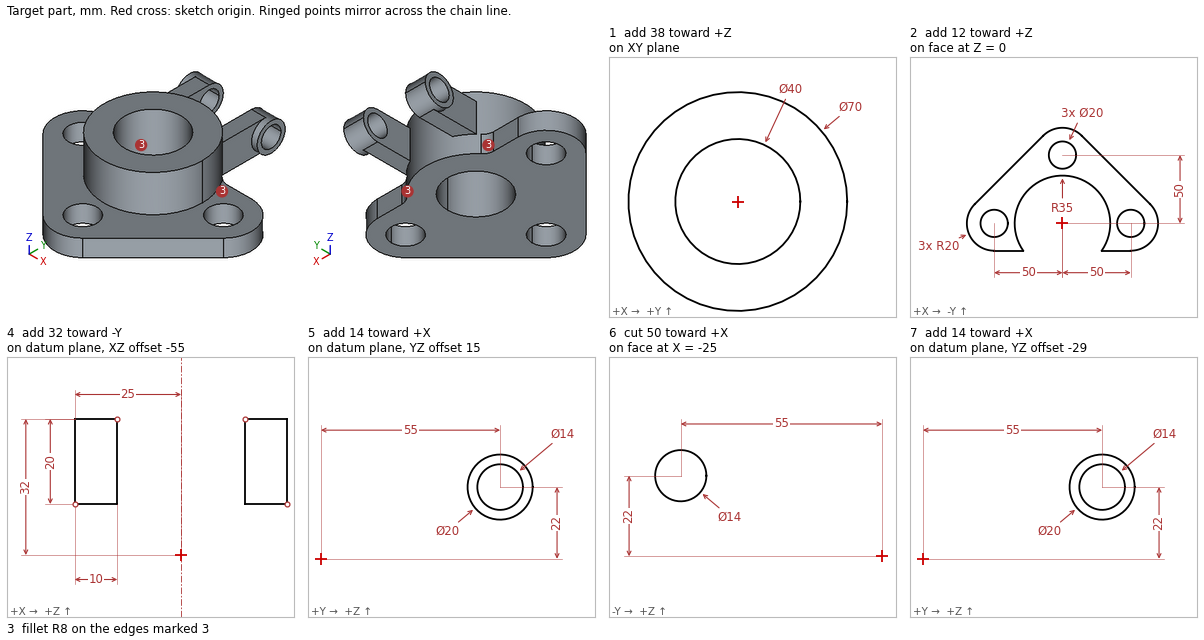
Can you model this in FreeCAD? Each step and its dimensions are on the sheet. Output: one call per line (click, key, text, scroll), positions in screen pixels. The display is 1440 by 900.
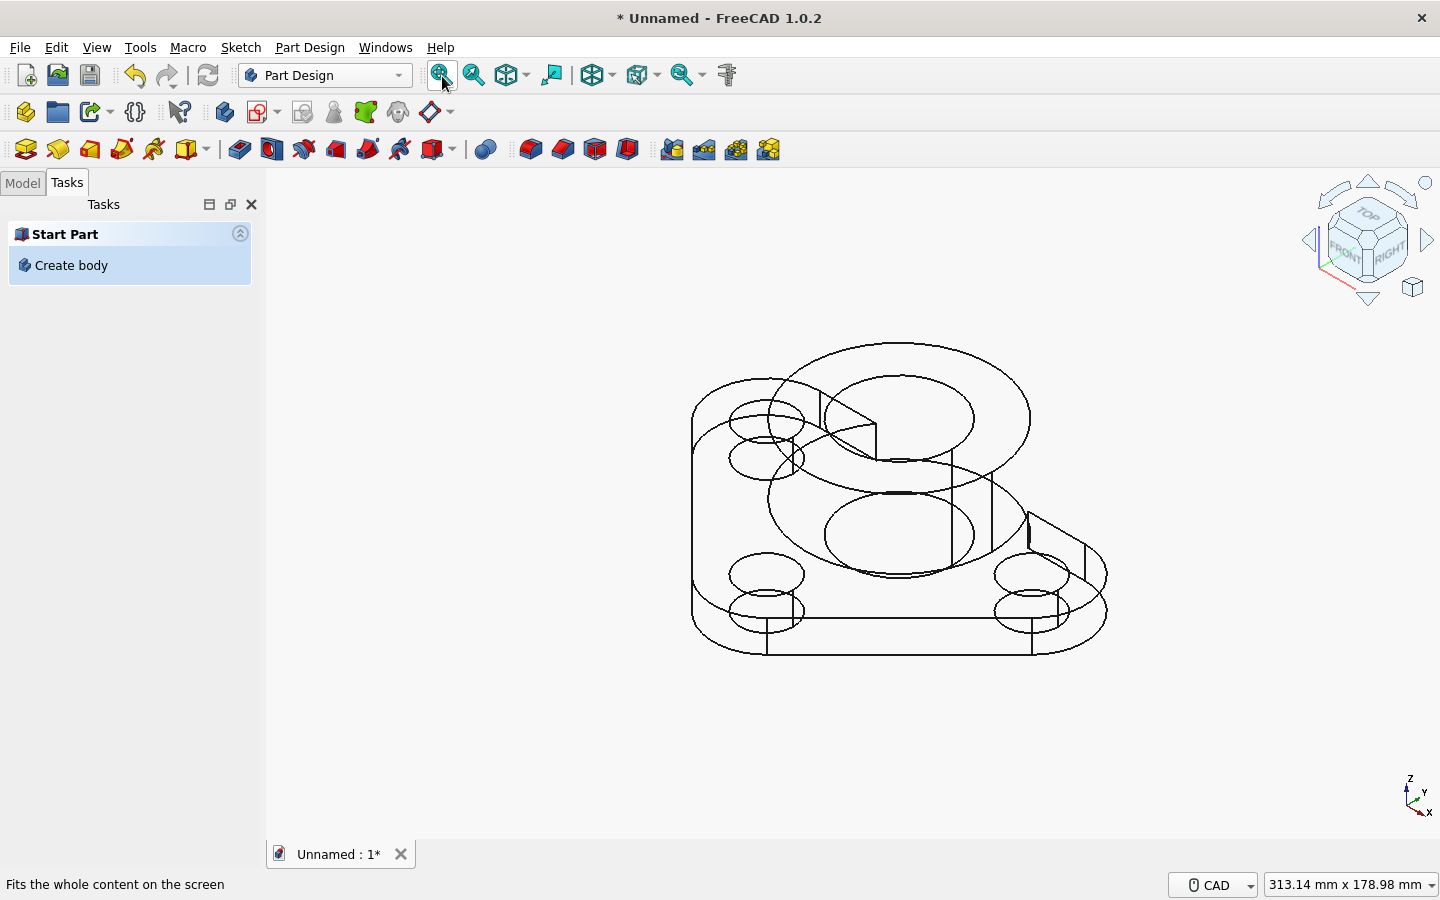
click(1028, 529)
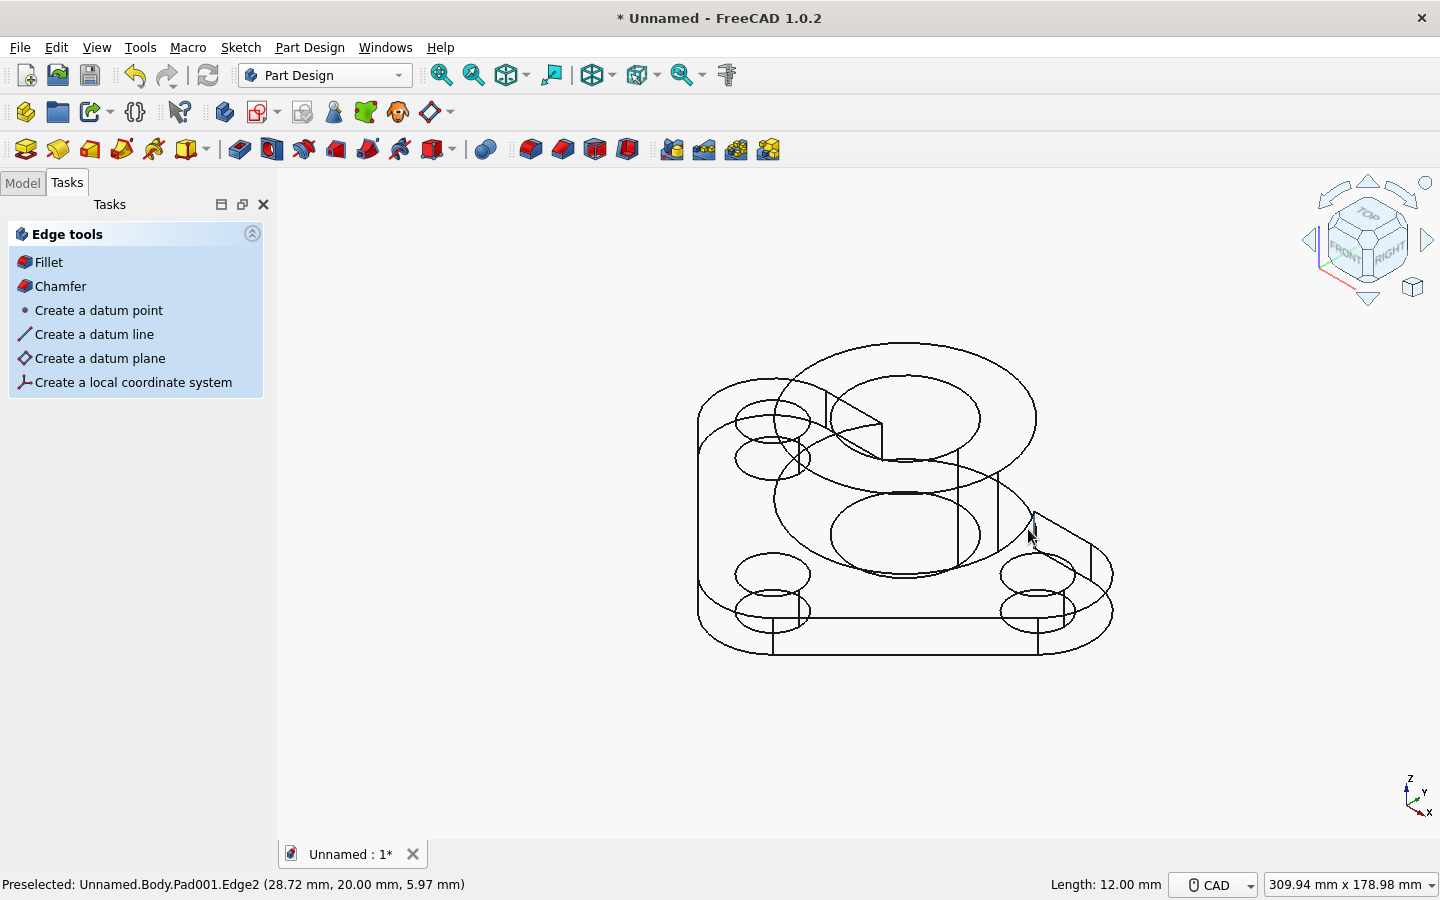
click(882, 441, ctrl)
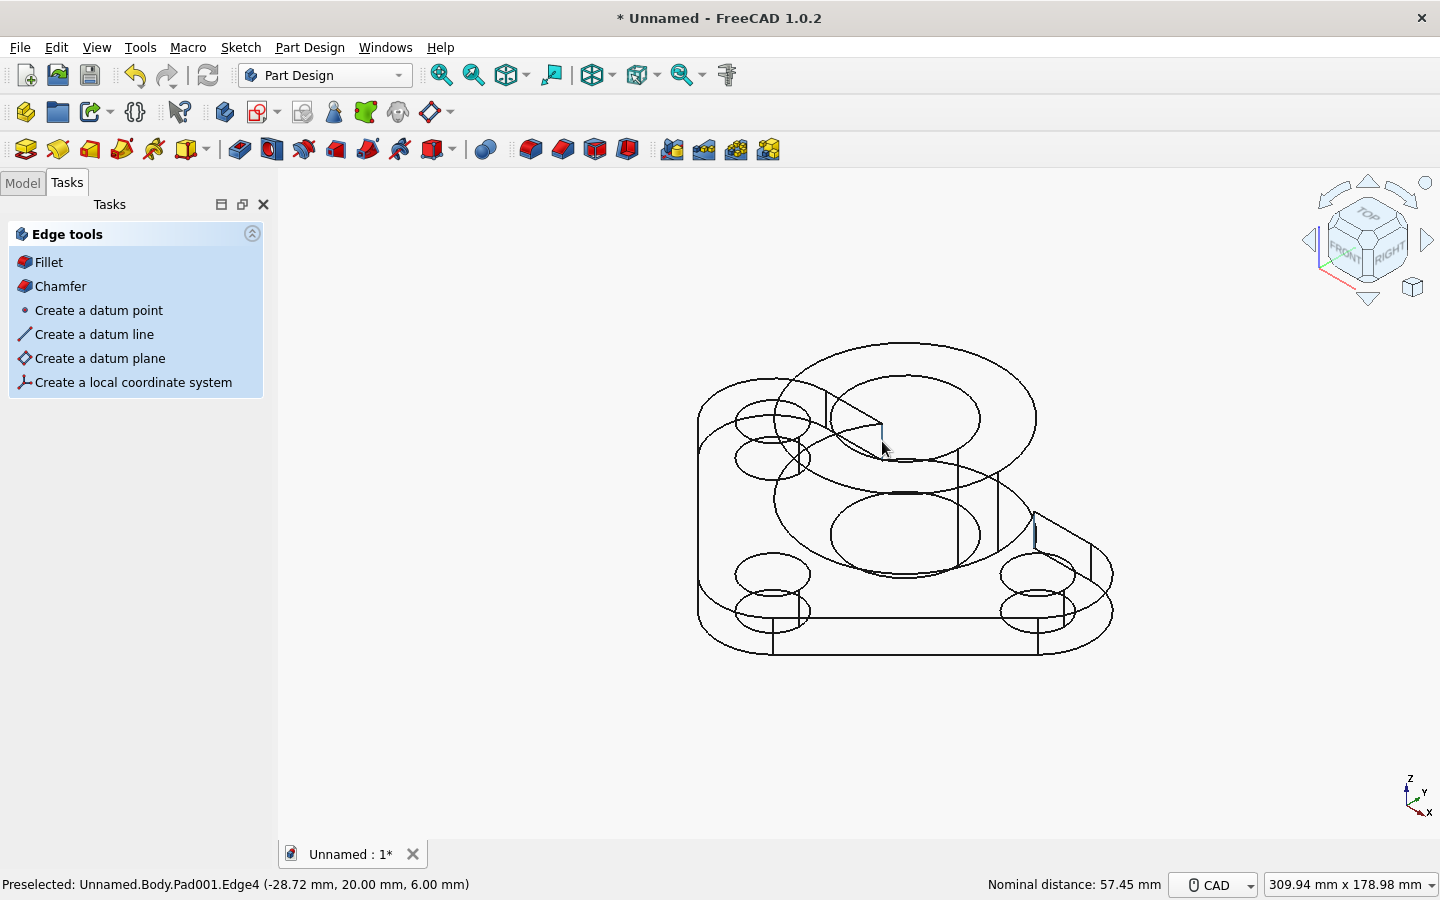
key(v)
key(1)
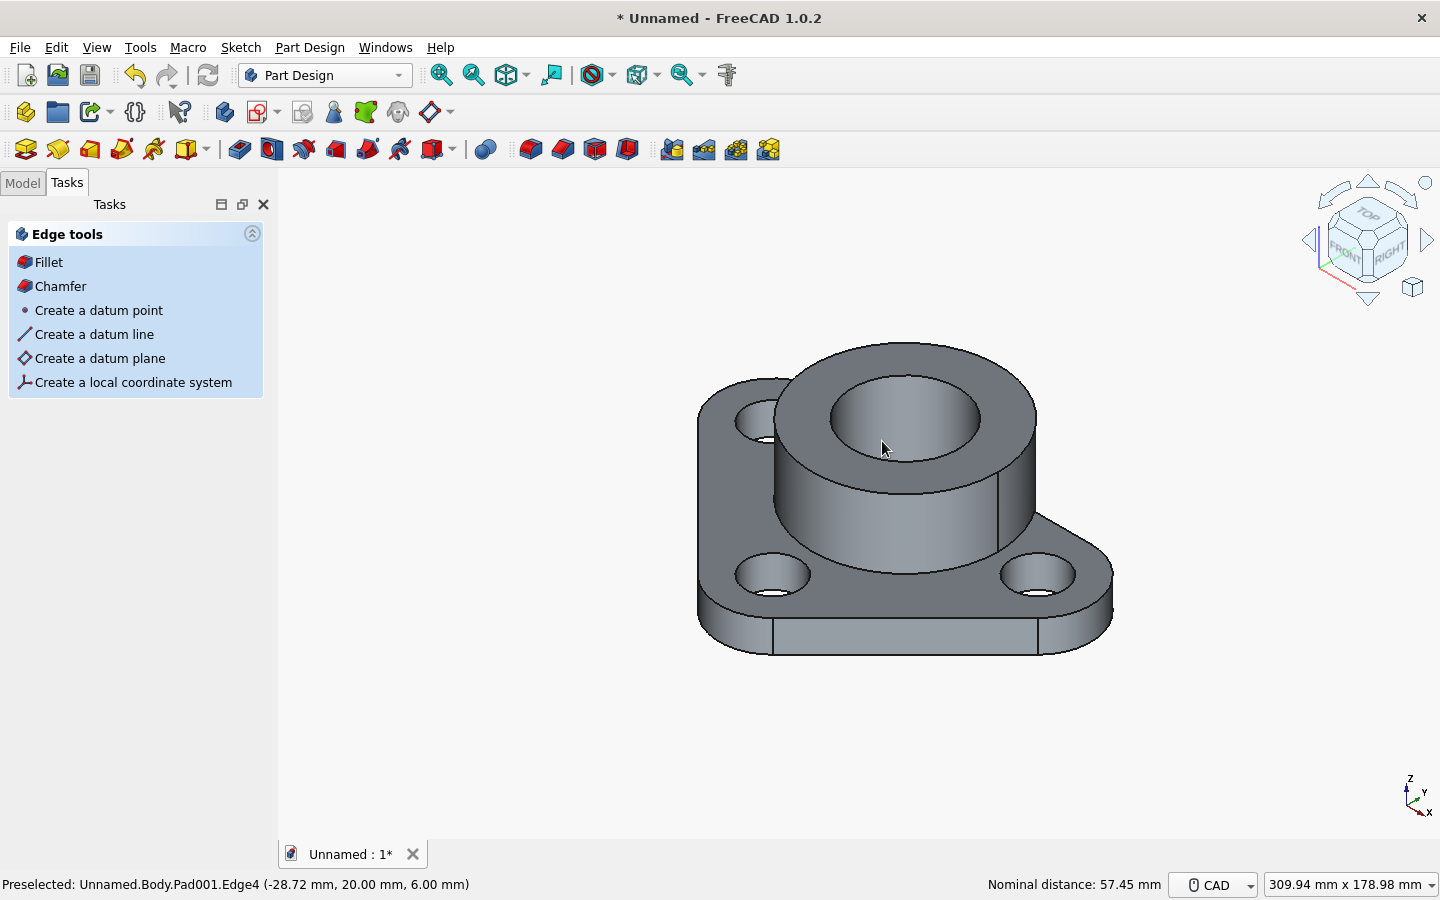
click(532, 150)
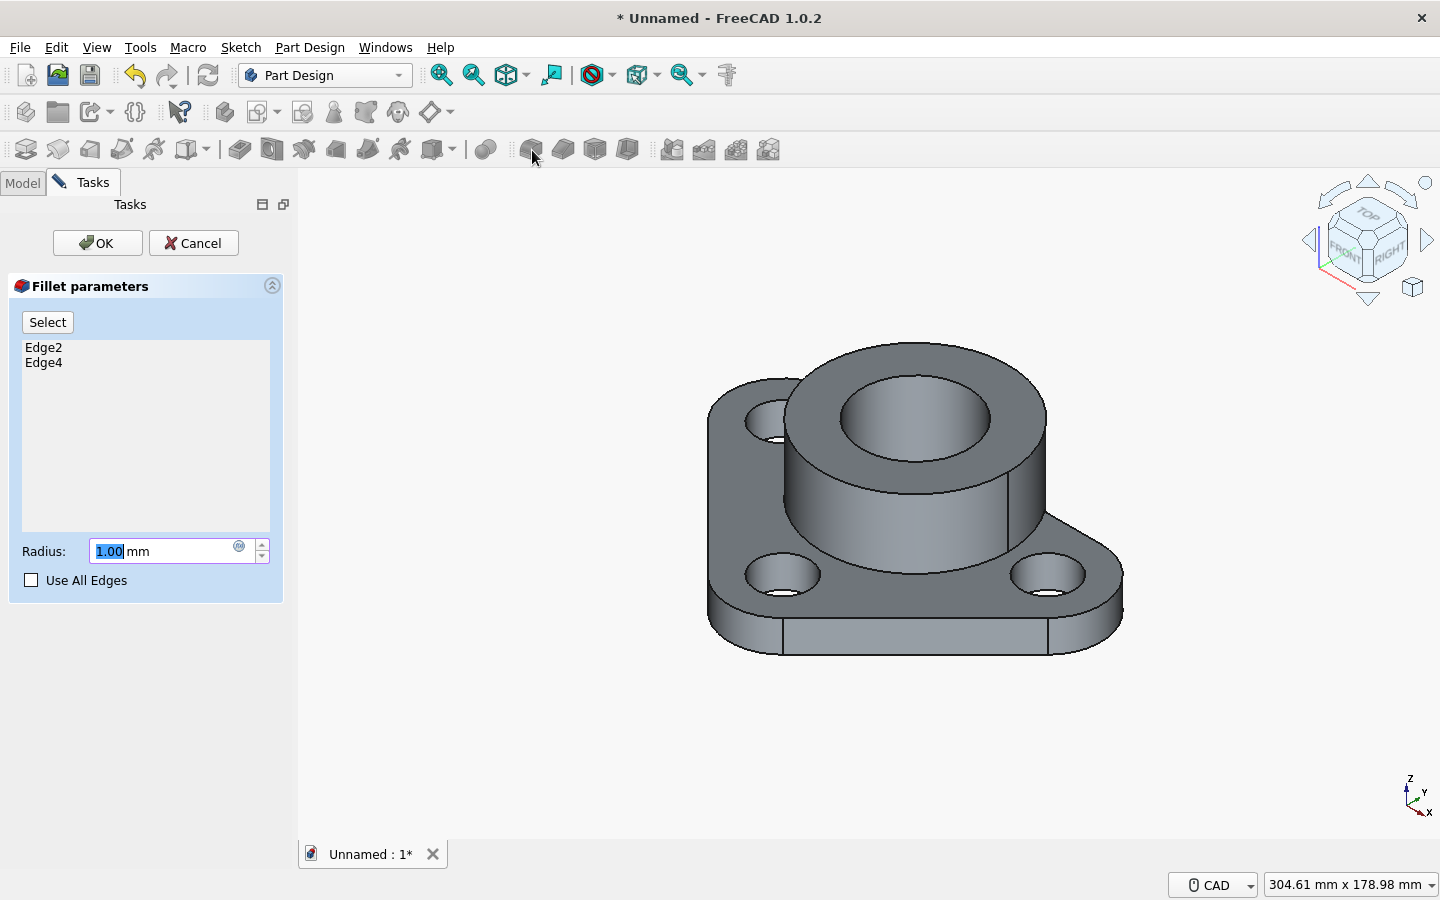
text(8)
key(Tab)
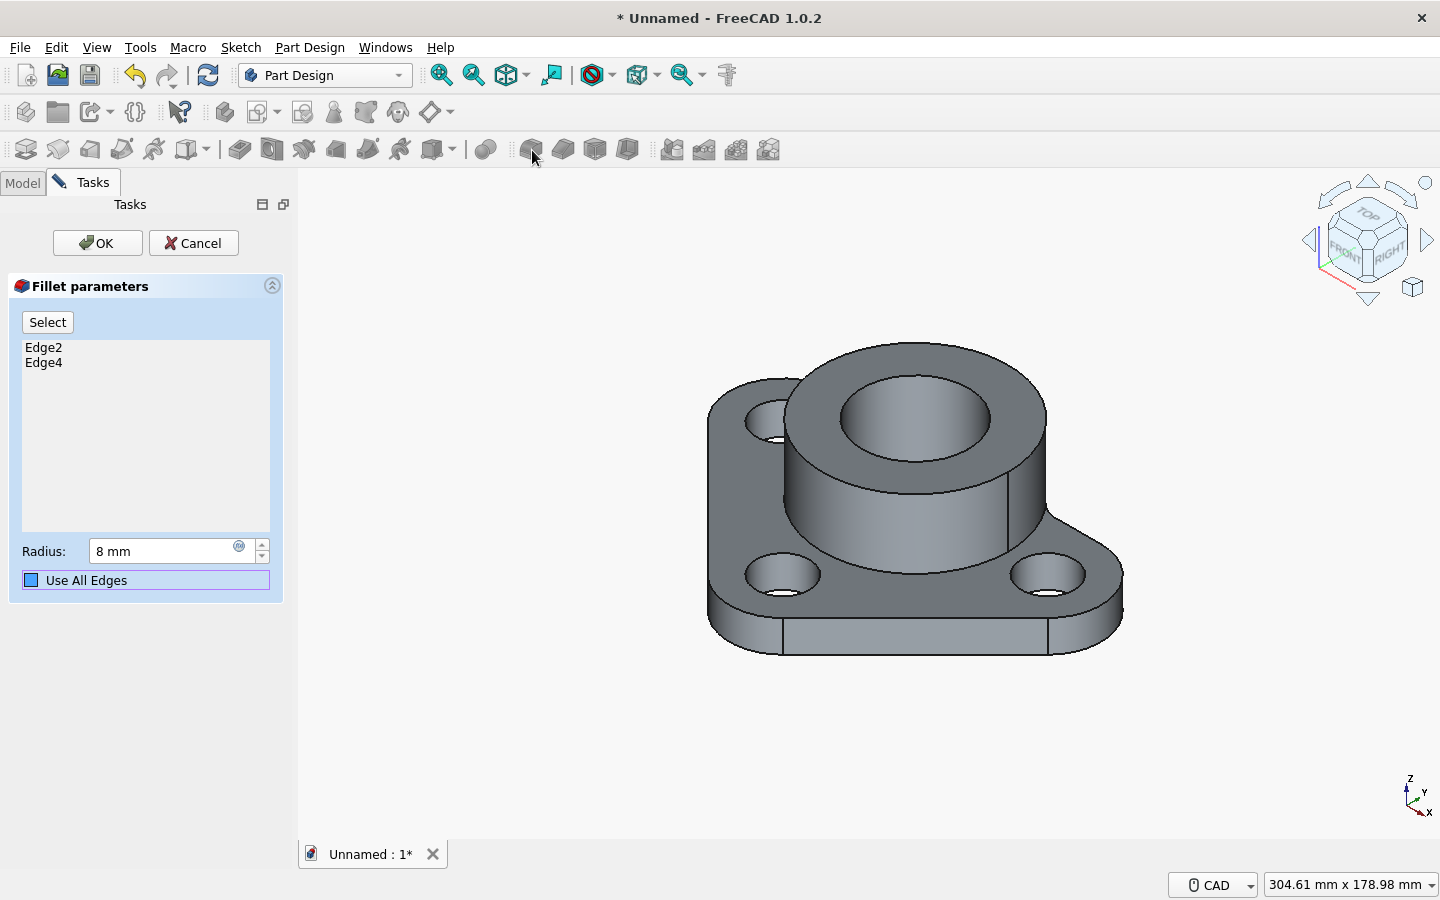
click(98, 243)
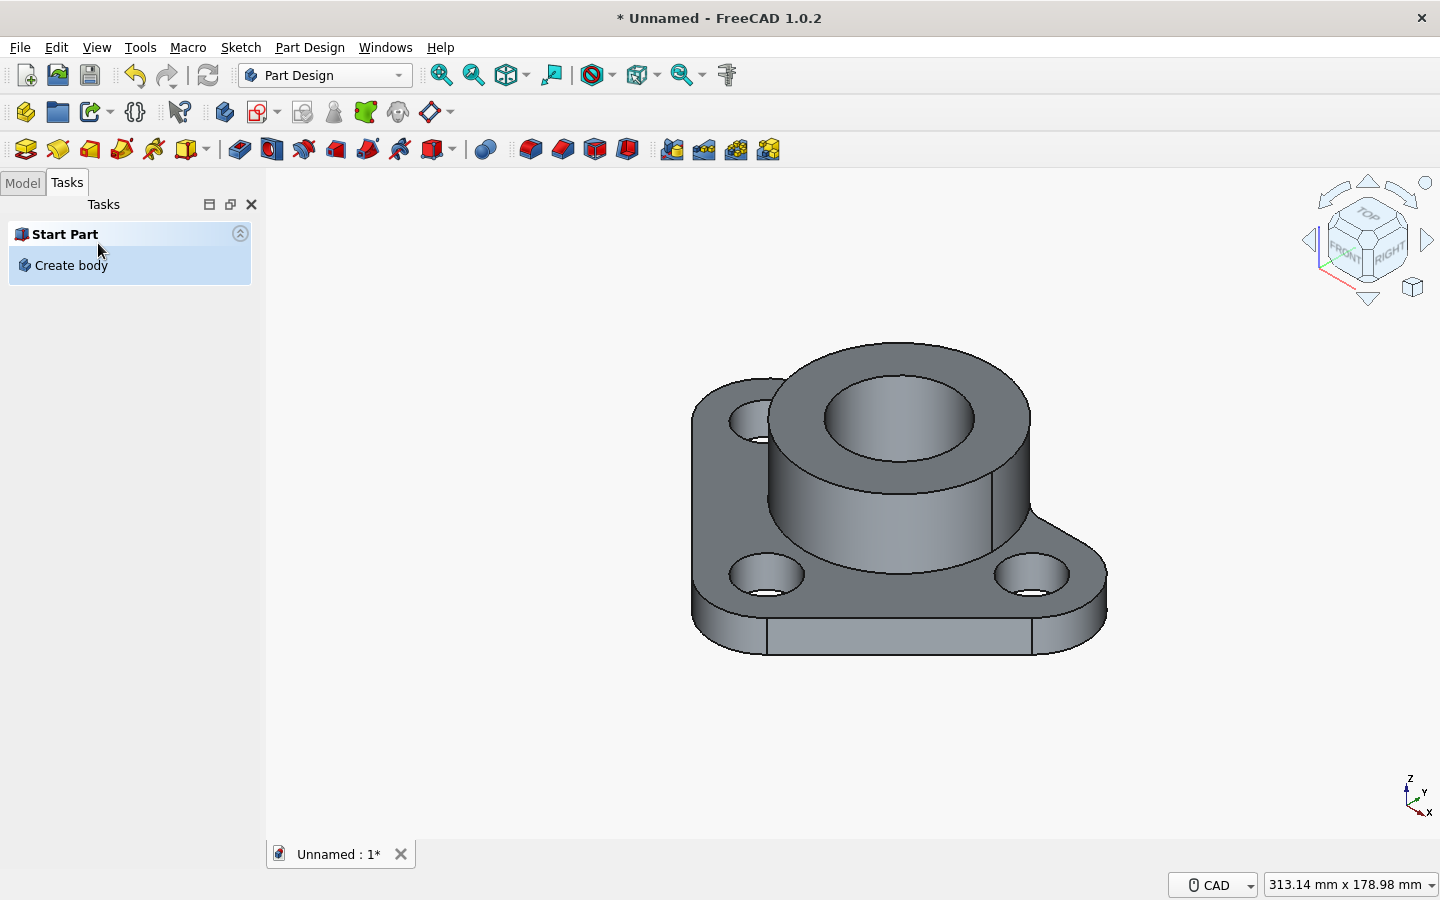
click(23, 182)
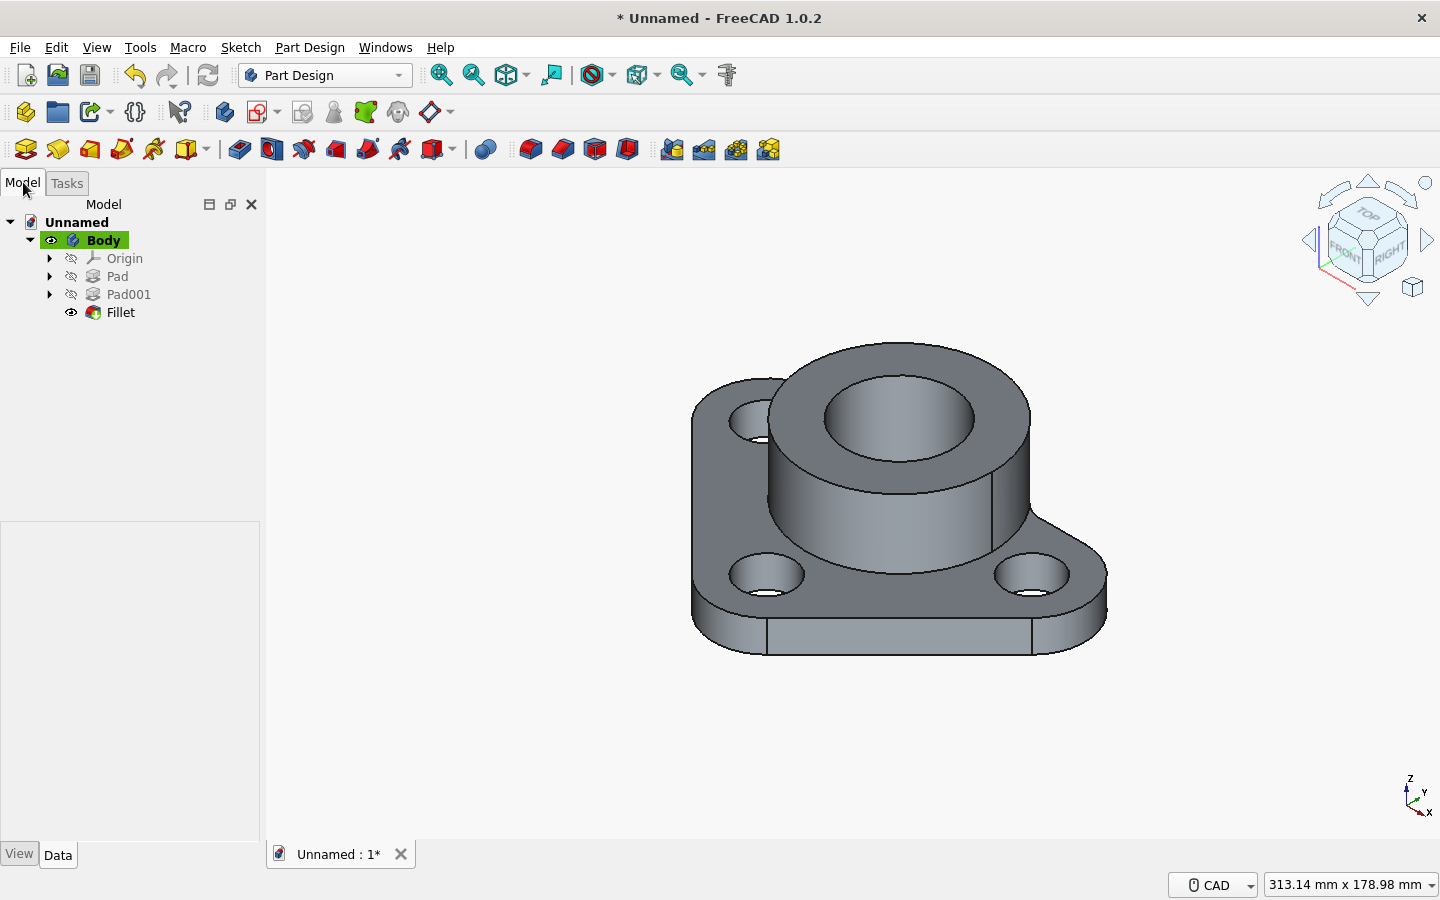
click(50, 258)